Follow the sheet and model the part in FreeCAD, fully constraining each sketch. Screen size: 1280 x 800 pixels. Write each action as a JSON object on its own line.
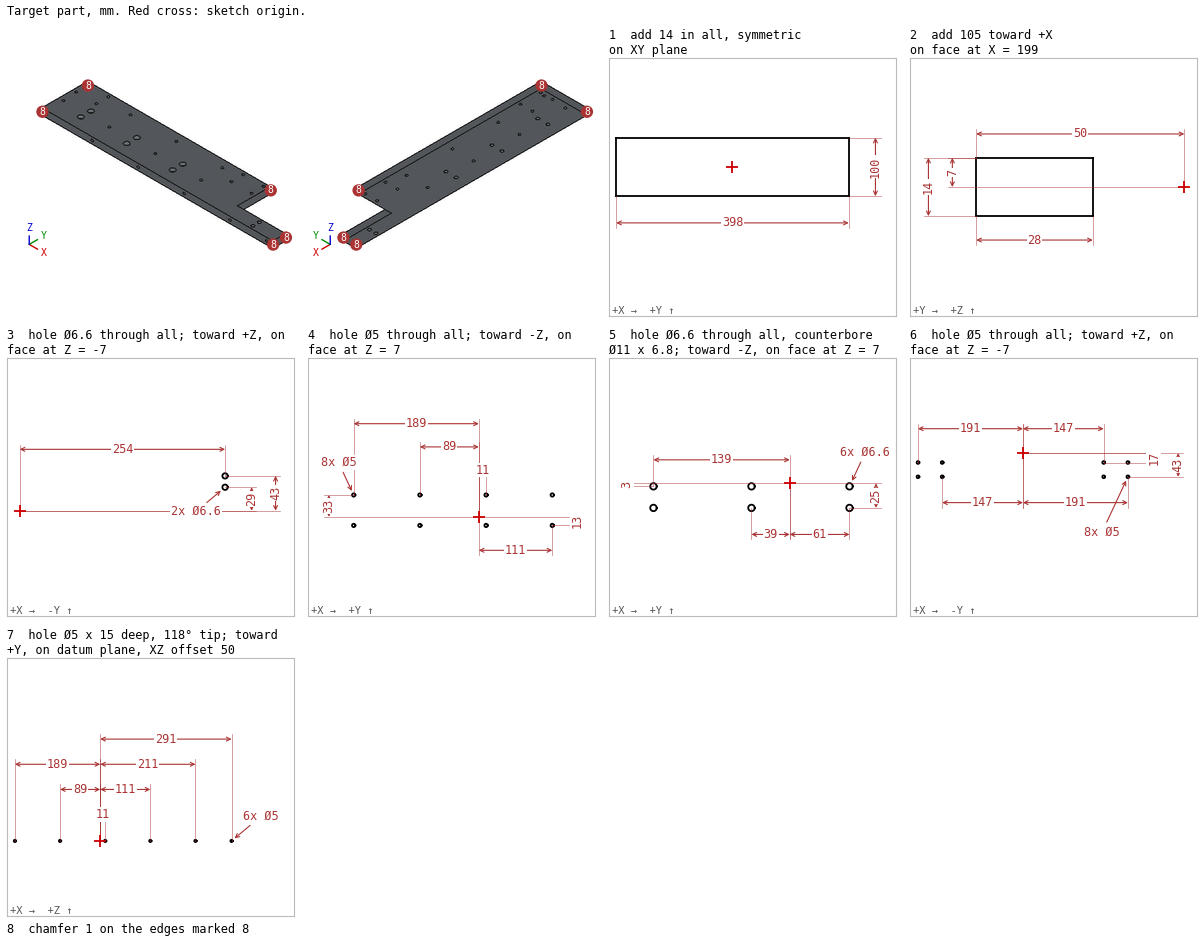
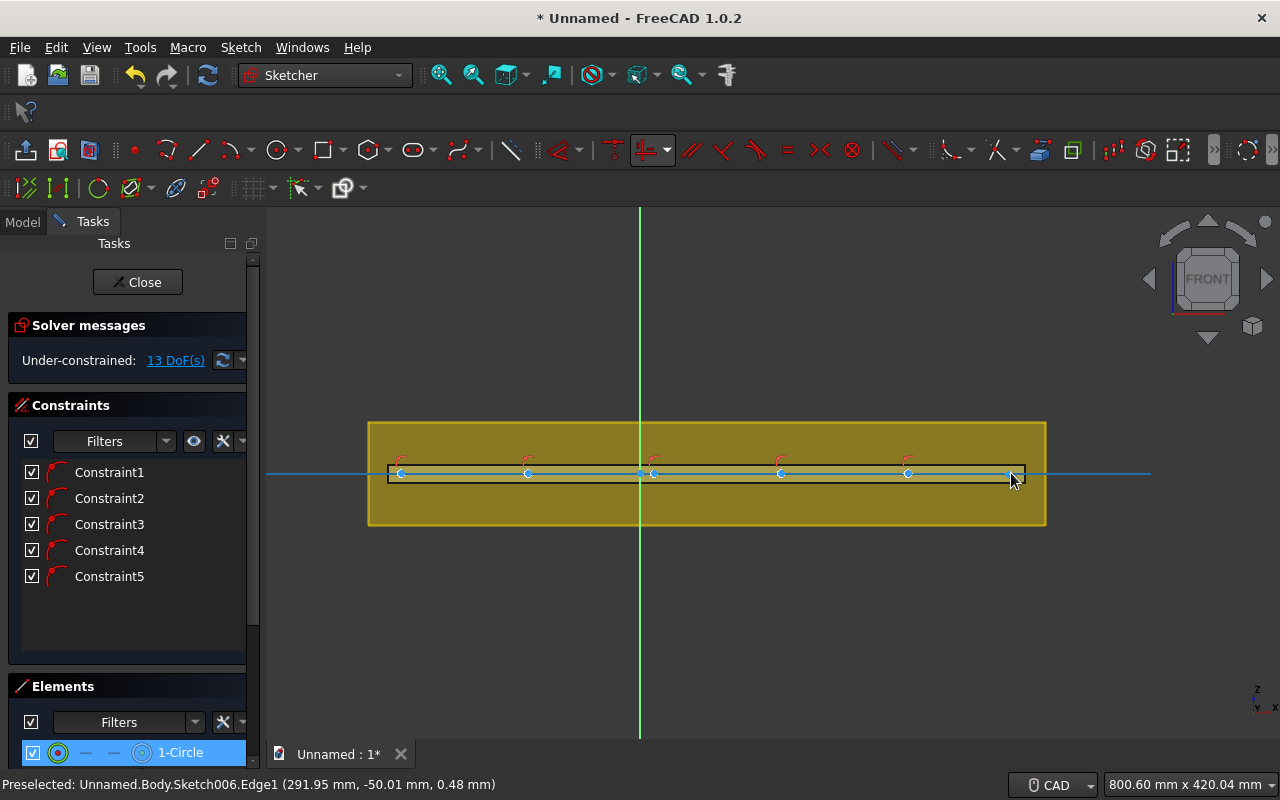
{"action": "scroll", "coordinate": [403, 471], "scroll_direction": "up", "scroll_amount": 9}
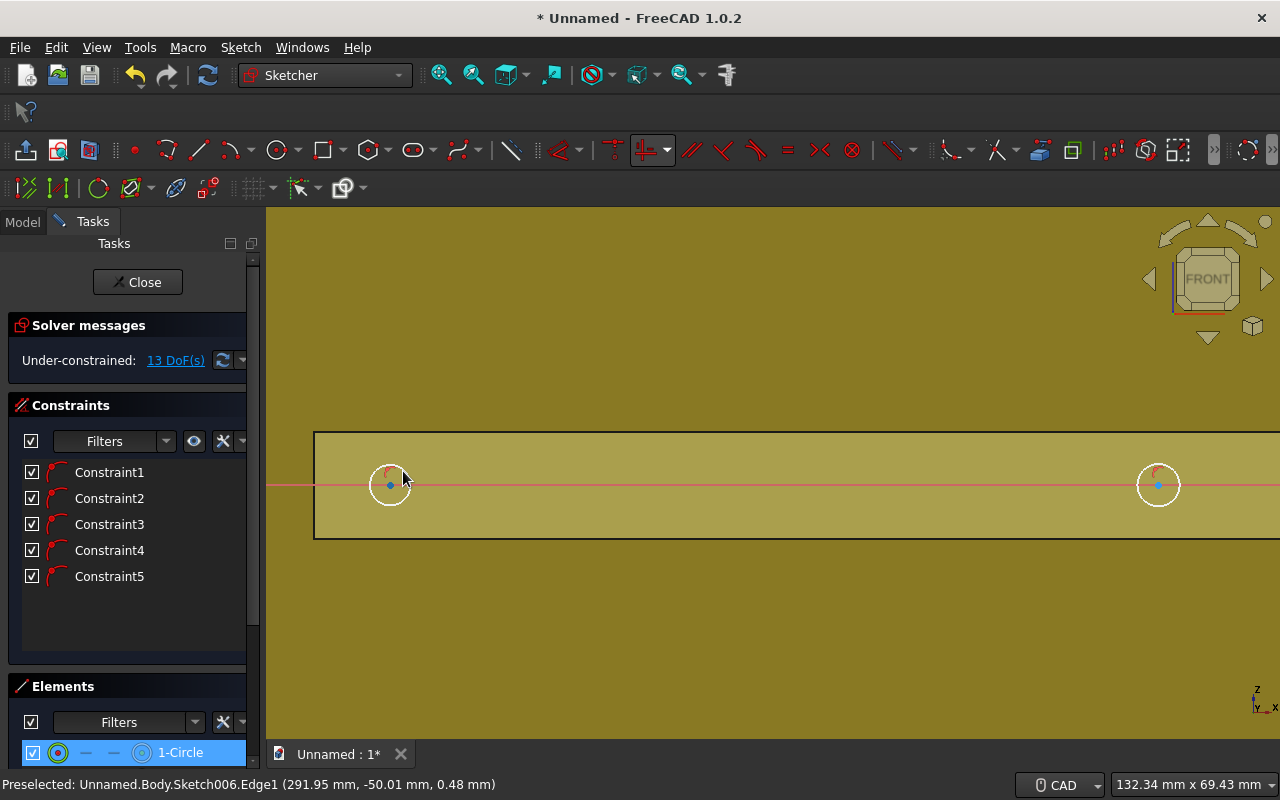
{"action": "left_click", "coordinate": [404, 471]}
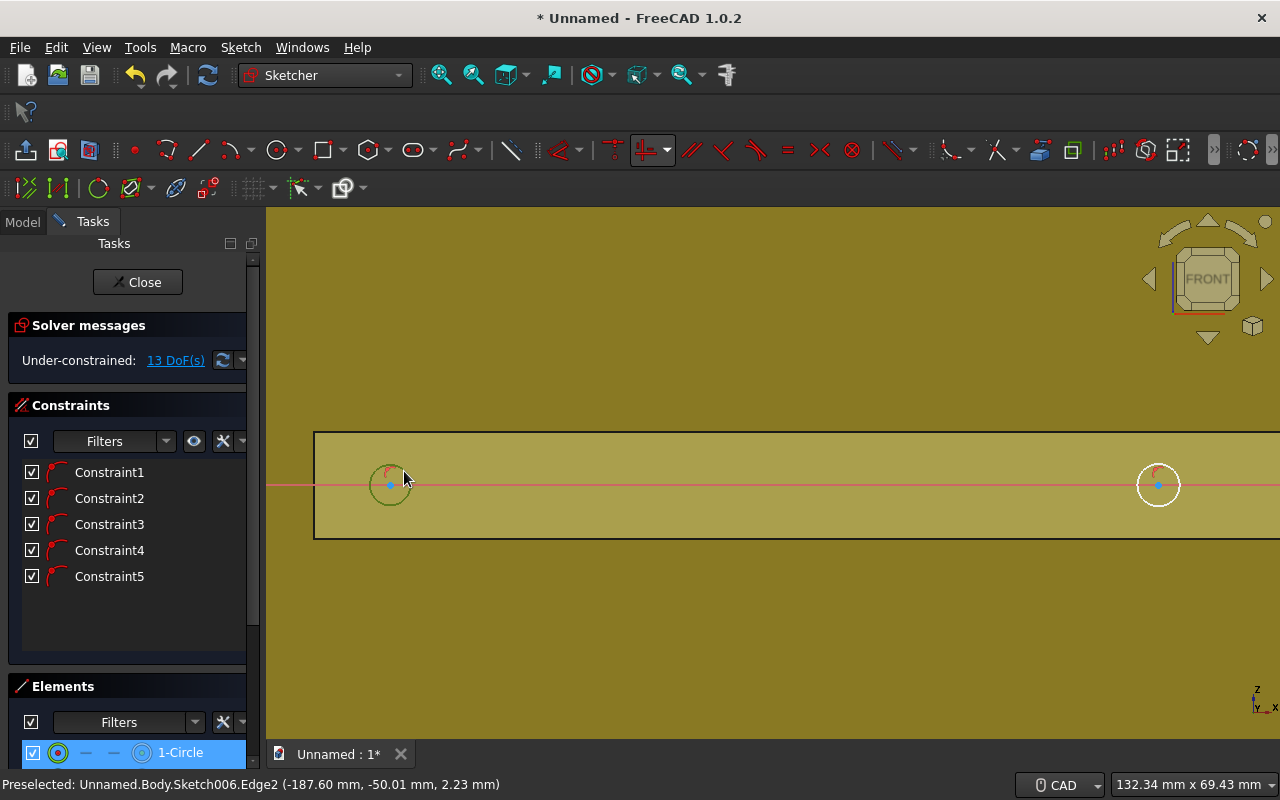
{"action": "scroll", "coordinate": [403, 471], "scroll_direction": "down", "scroll_amount": 9}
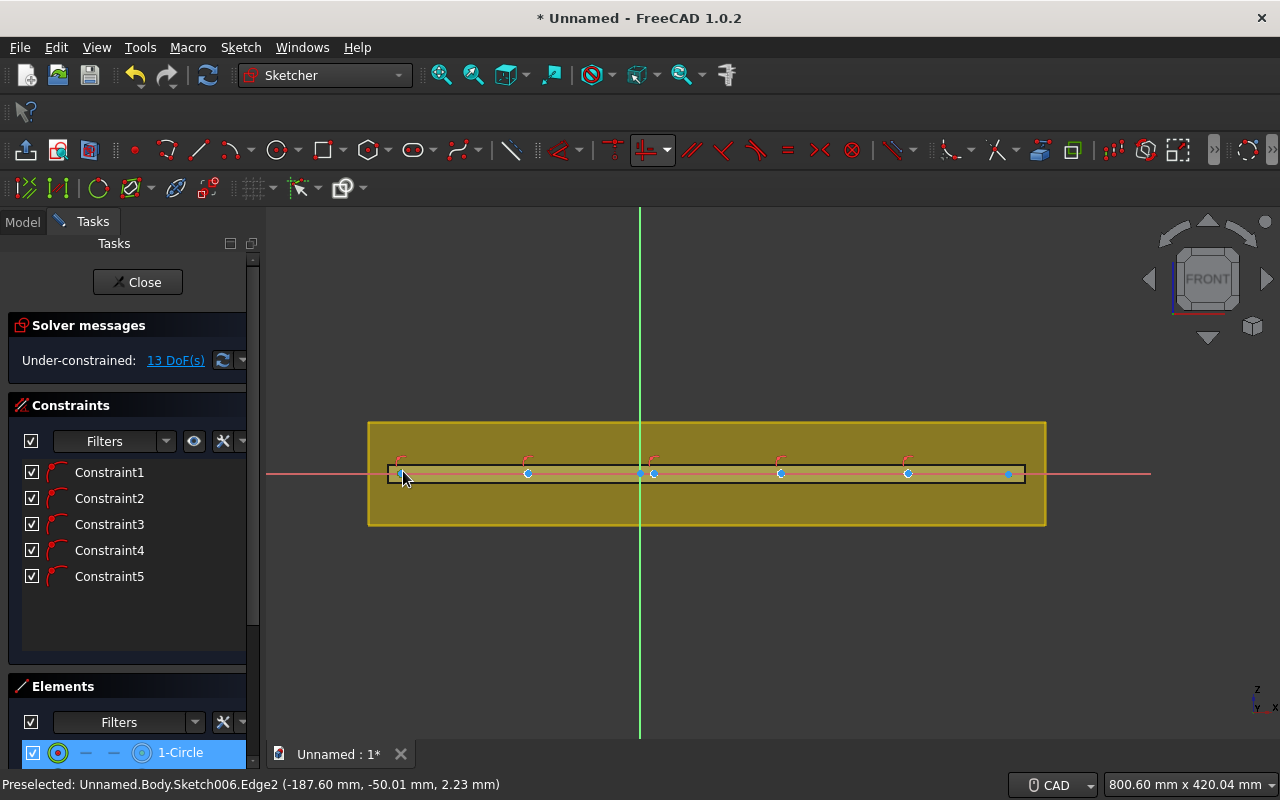
{"action": "scroll", "coordinate": [530, 471], "scroll_direction": "up", "scroll_amount": 9}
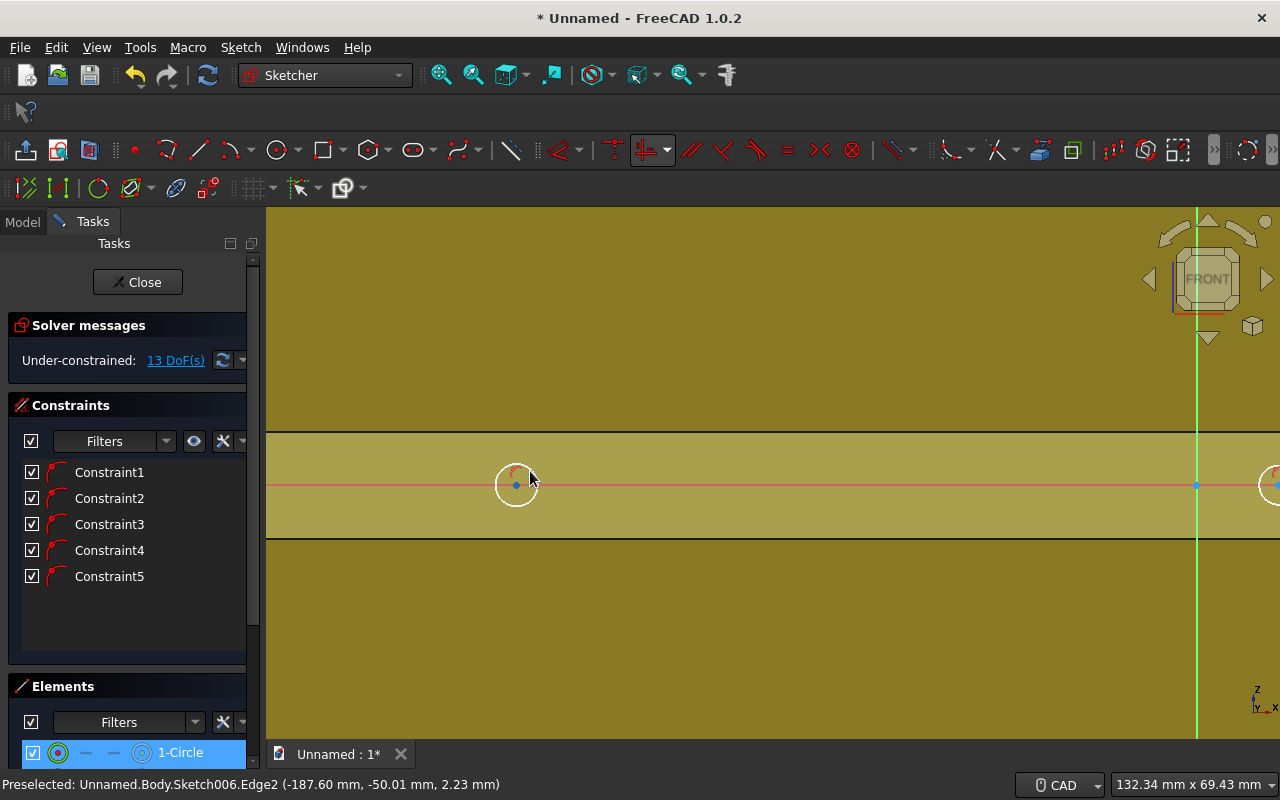
{"action": "left_click", "coordinate": [531, 470]}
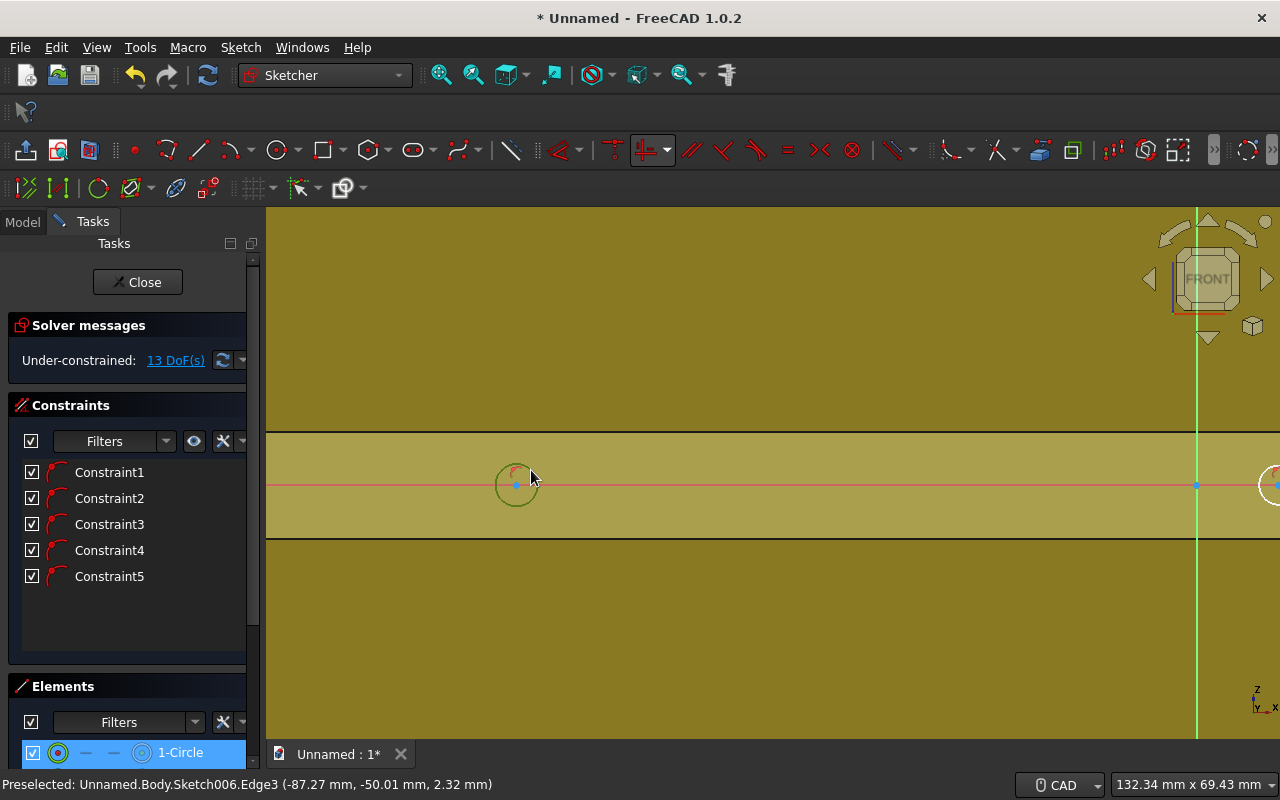
{"action": "scroll", "coordinate": [530, 471], "scroll_direction": "down", "scroll_amount": 9}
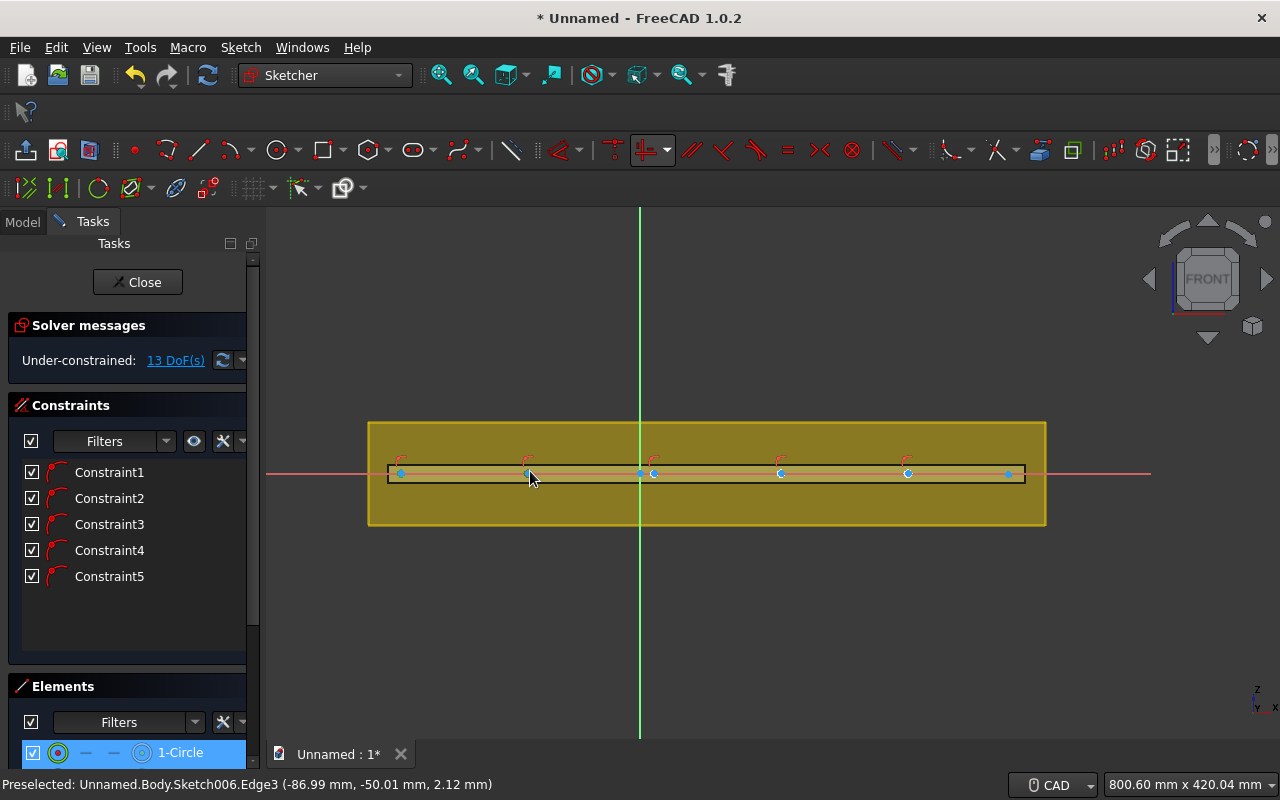
{"action": "scroll", "coordinate": [656, 471], "scroll_direction": "up", "scroll_amount": 9}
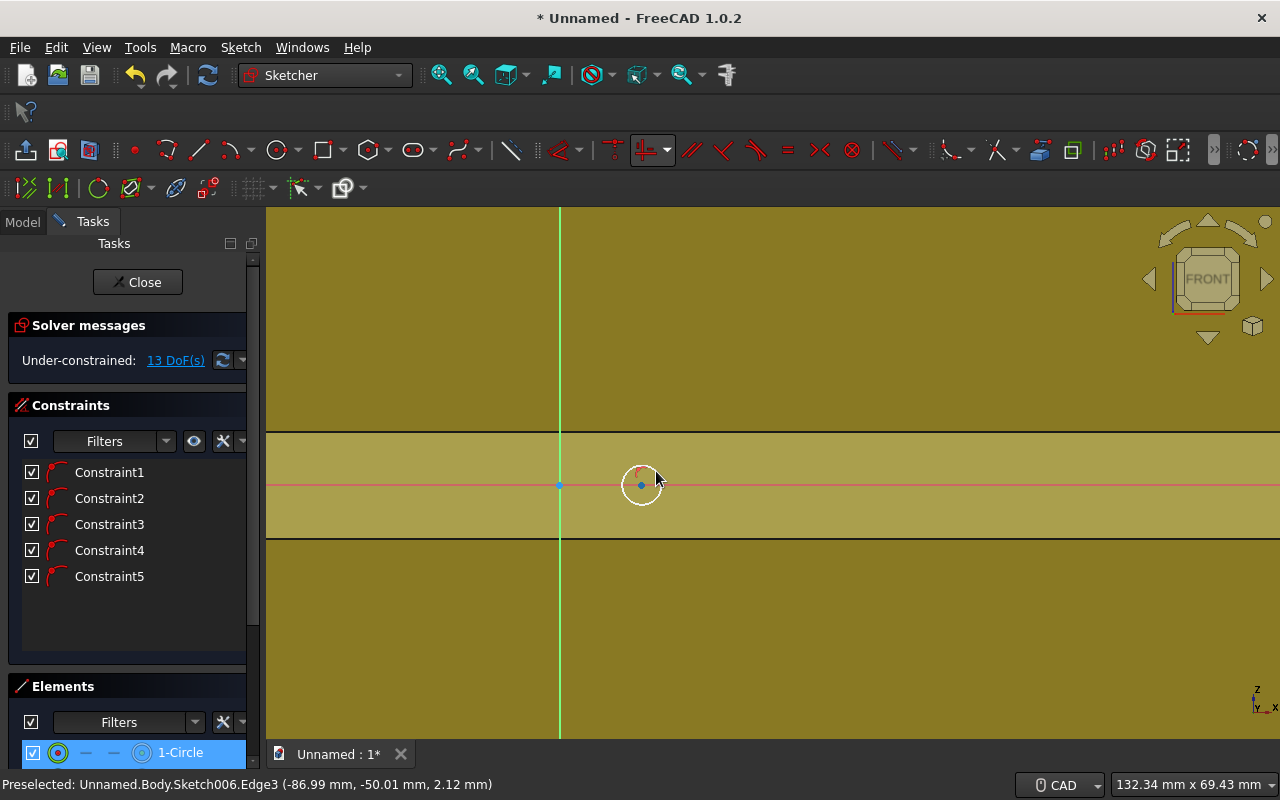
{"action": "left_click", "coordinate": [656, 471]}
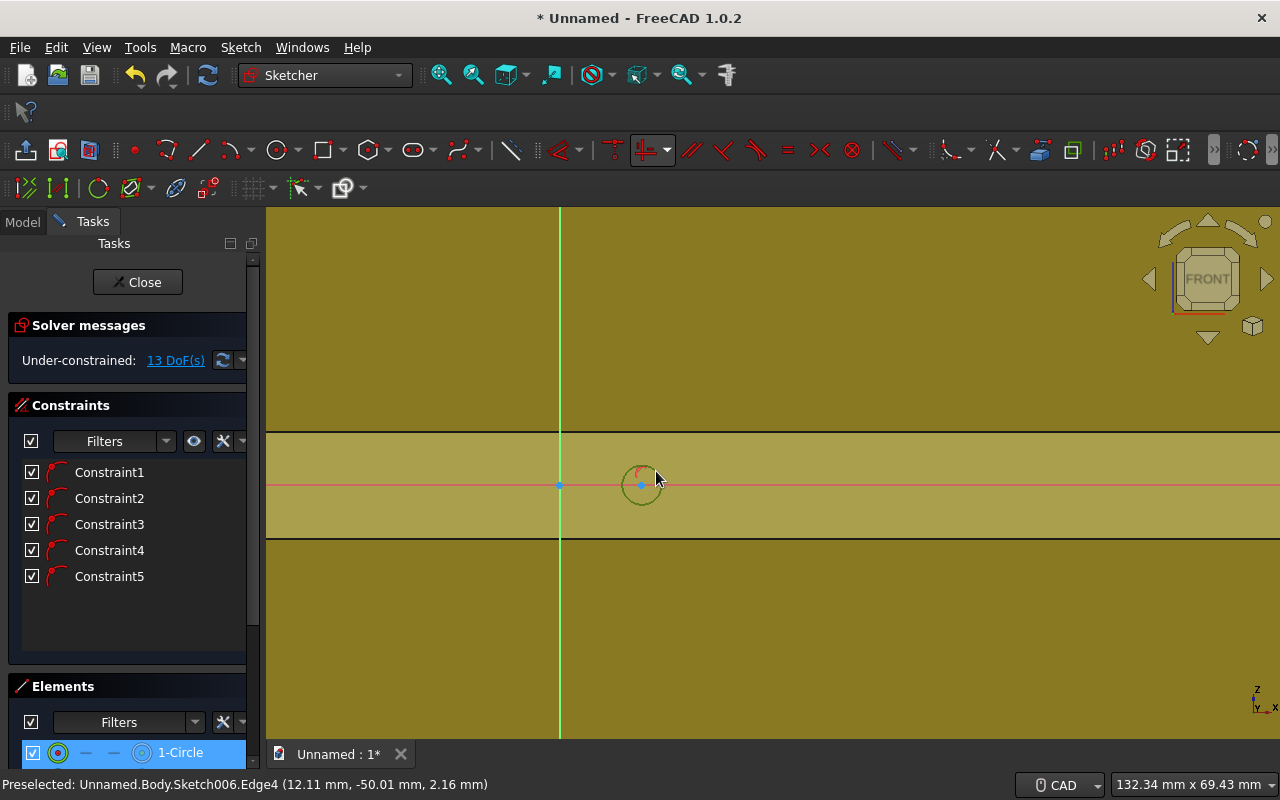
{"action": "scroll", "coordinate": [656, 471], "scroll_direction": "down", "scroll_amount": 9}